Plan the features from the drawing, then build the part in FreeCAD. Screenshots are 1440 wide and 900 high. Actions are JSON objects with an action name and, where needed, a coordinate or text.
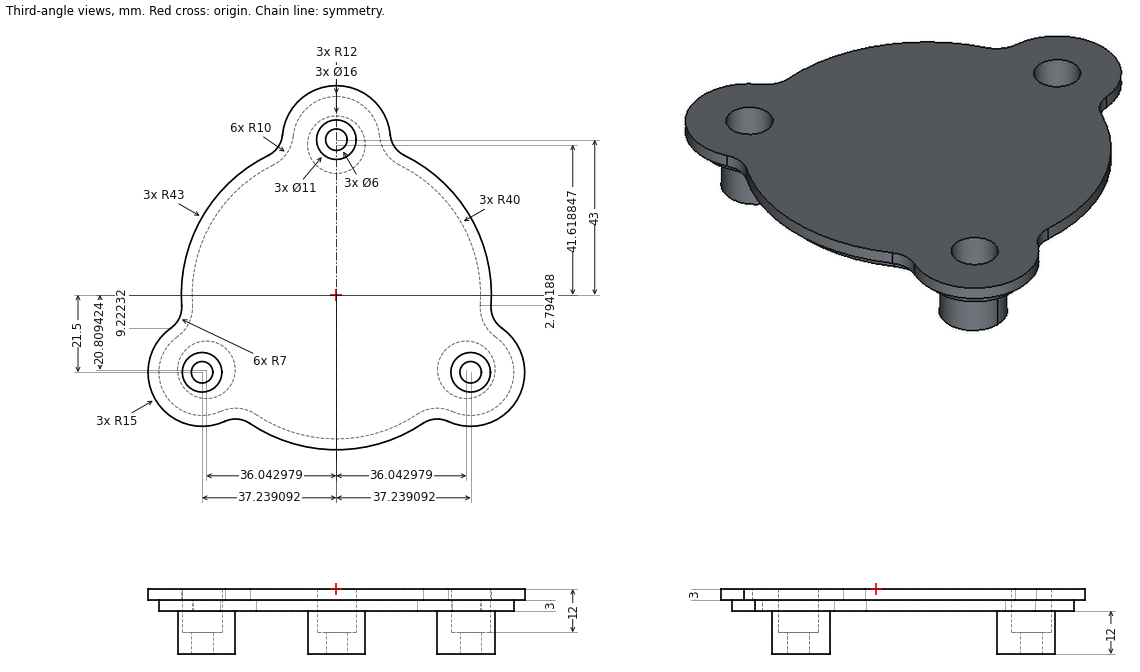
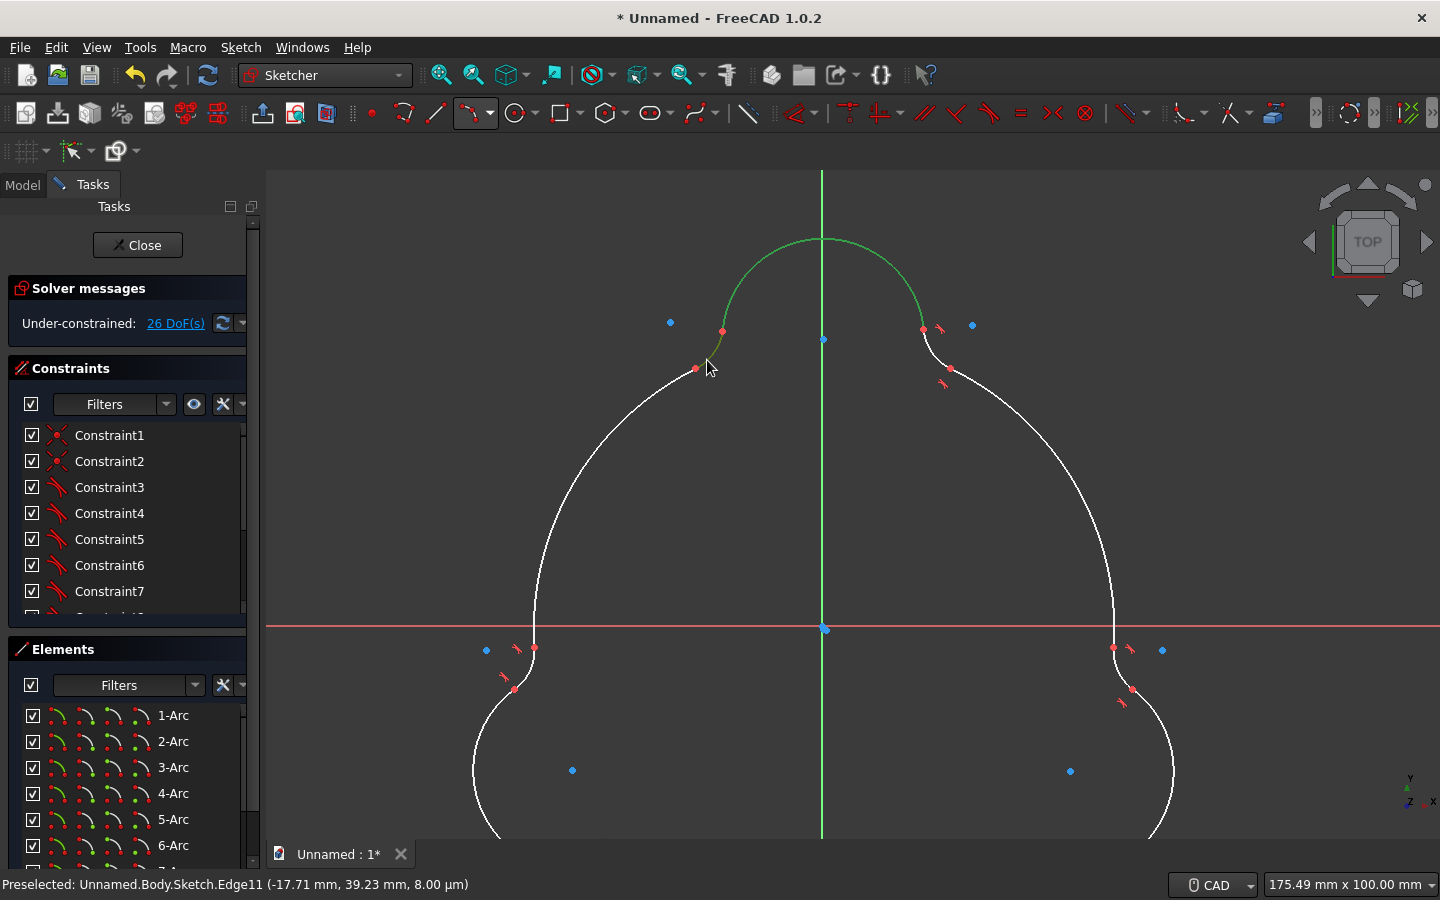
{"action": "left_click", "coordinate": [990, 114]}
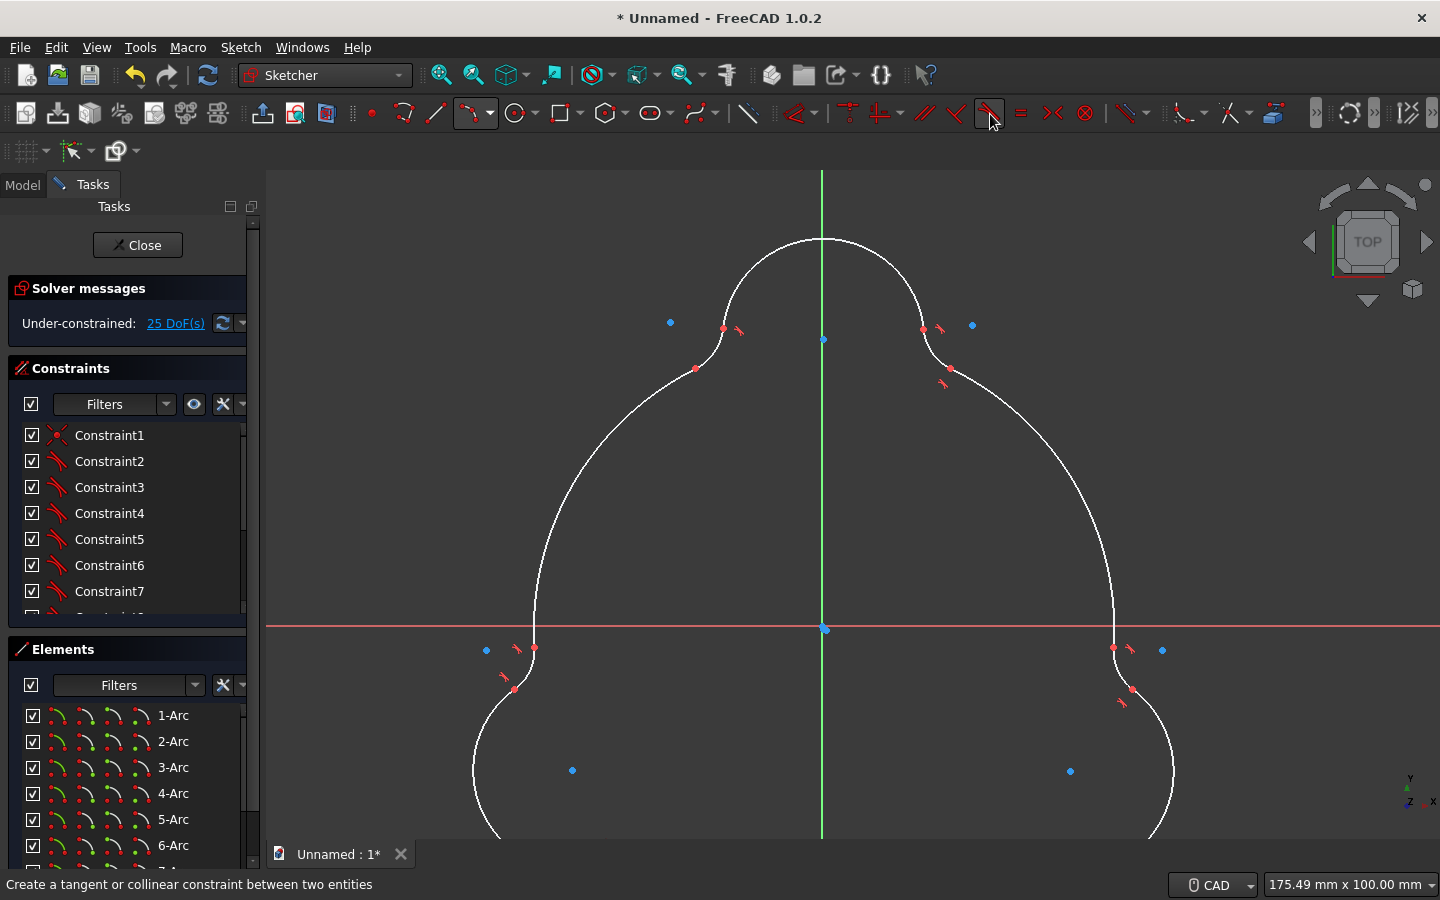
{"action": "left_click", "coordinate": [708, 360]}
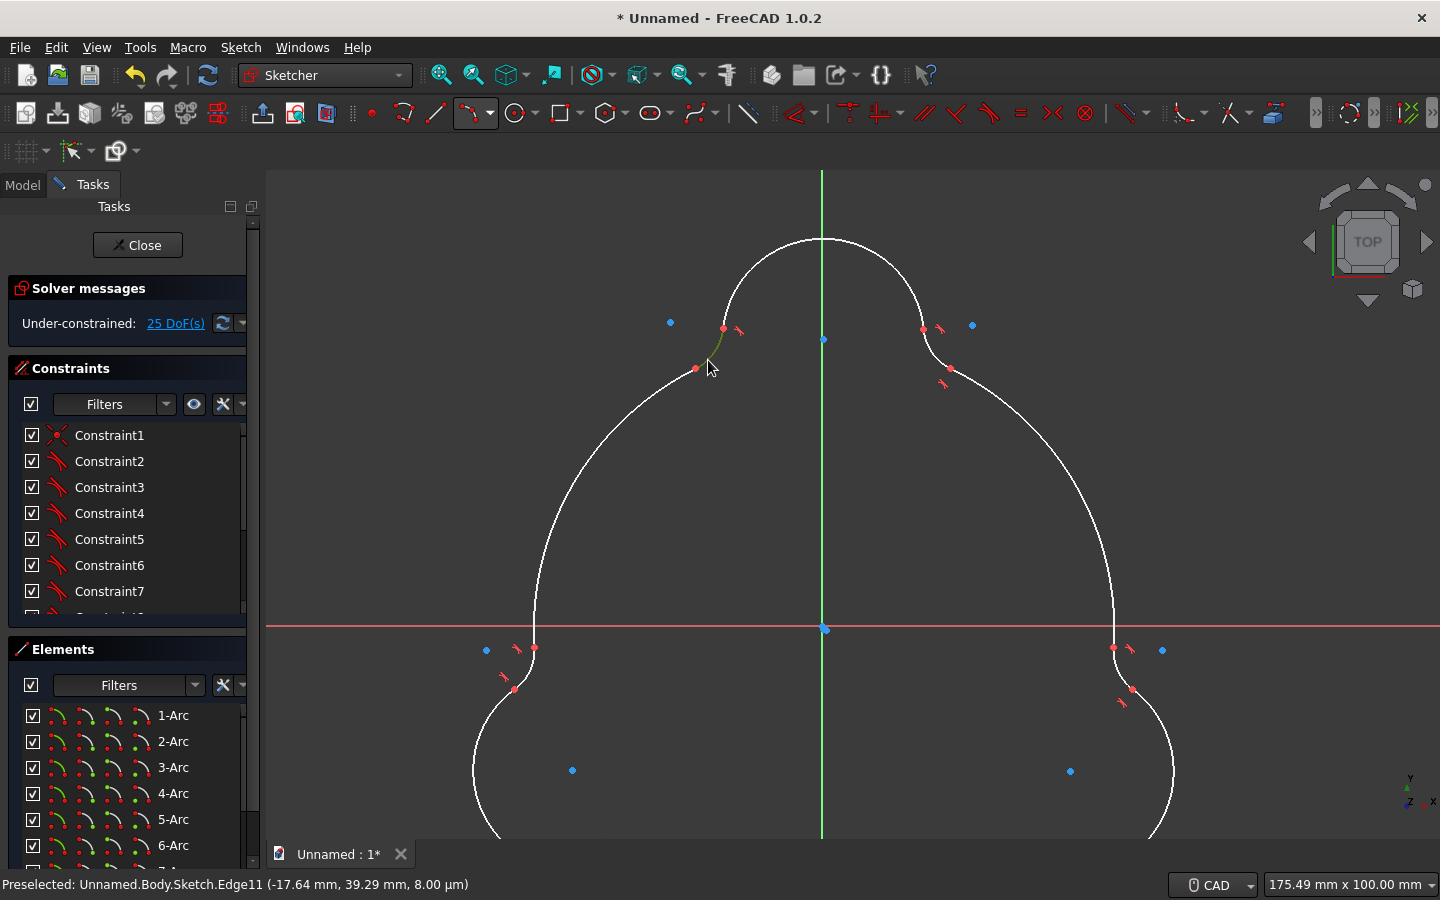
{"action": "left_click", "coordinate": [614, 429]}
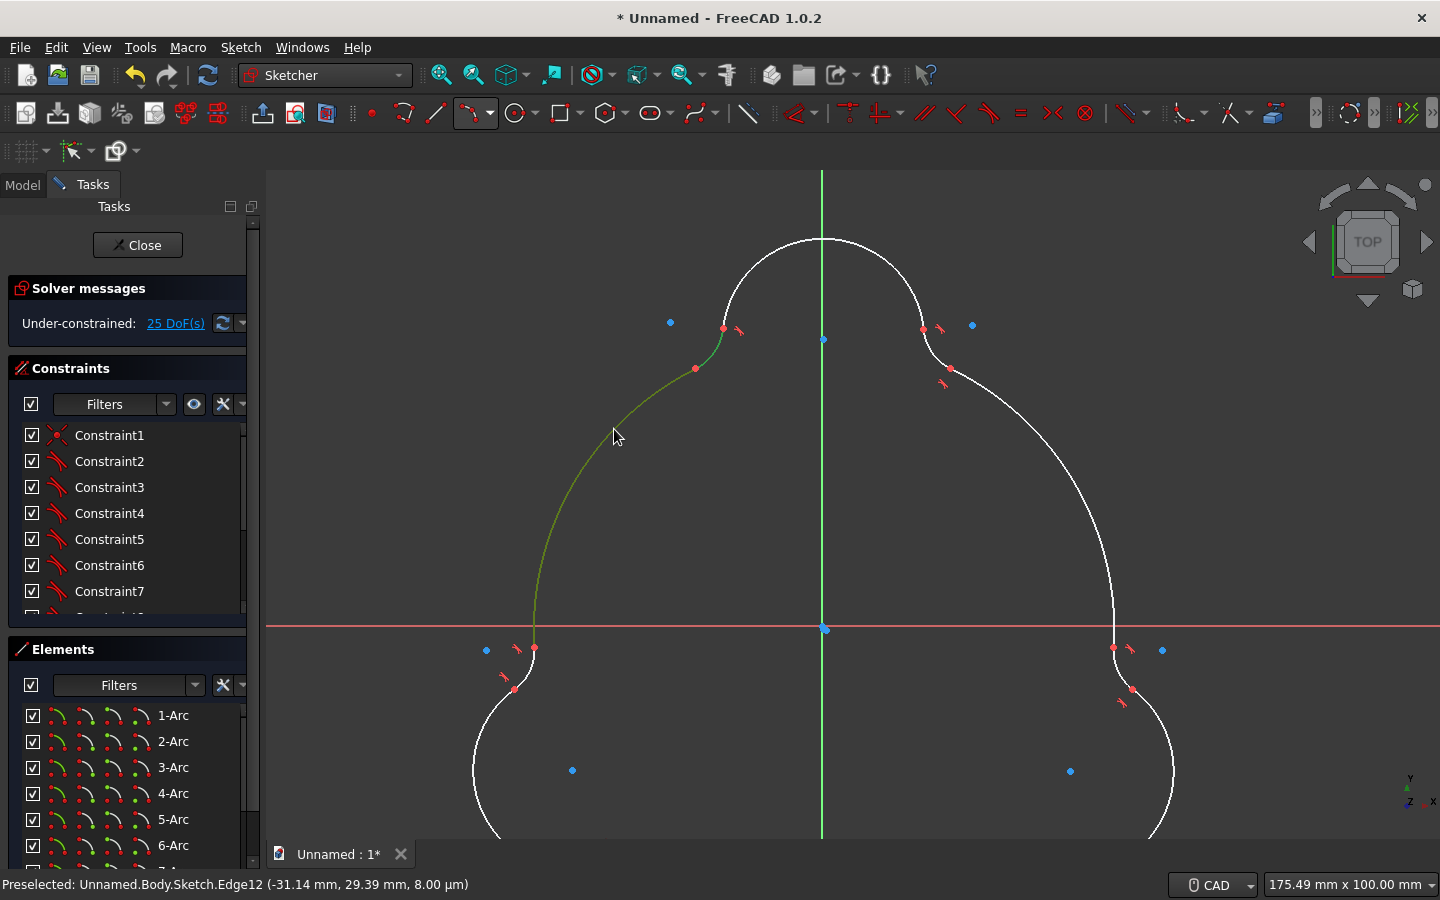
{"action": "left_click", "coordinate": [990, 114]}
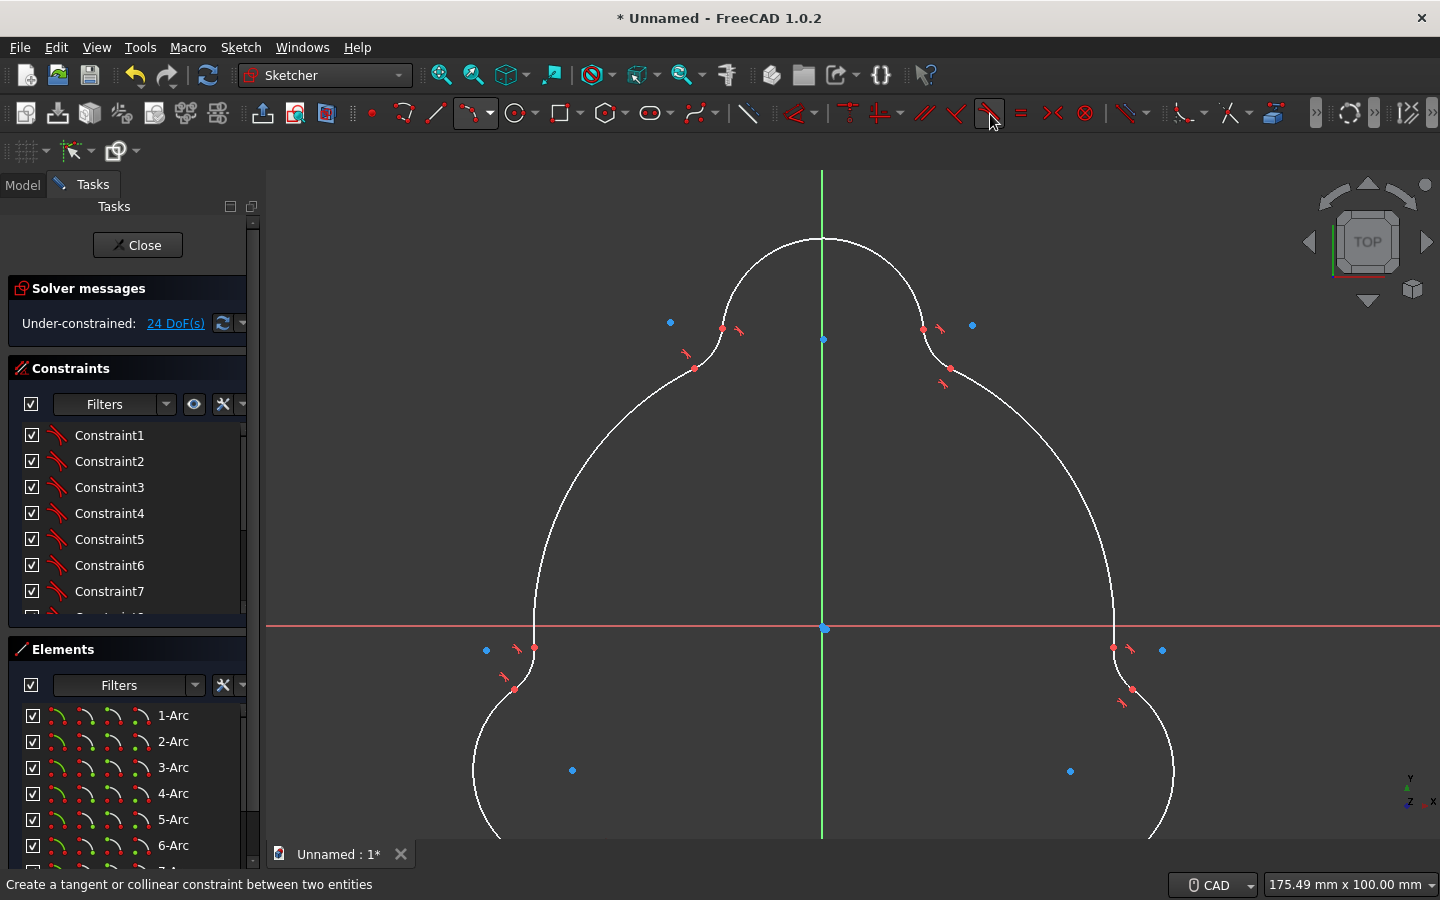
{"action": "scroll", "coordinate": [708, 359], "scroll_direction": "down", "scroll_amount": 2}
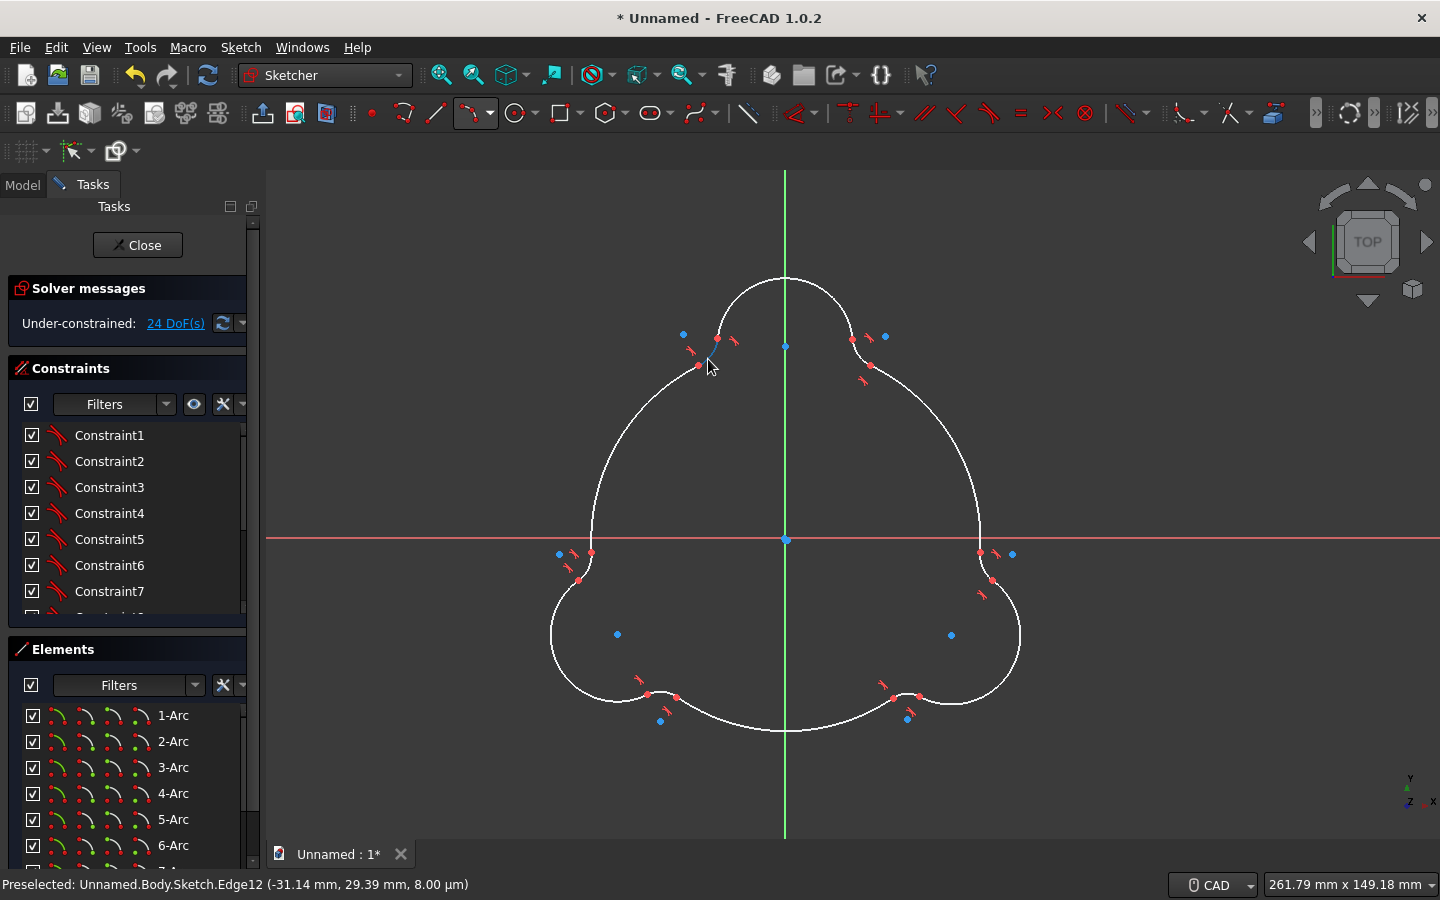
{"action": "left_click", "coordinate": [739, 725]}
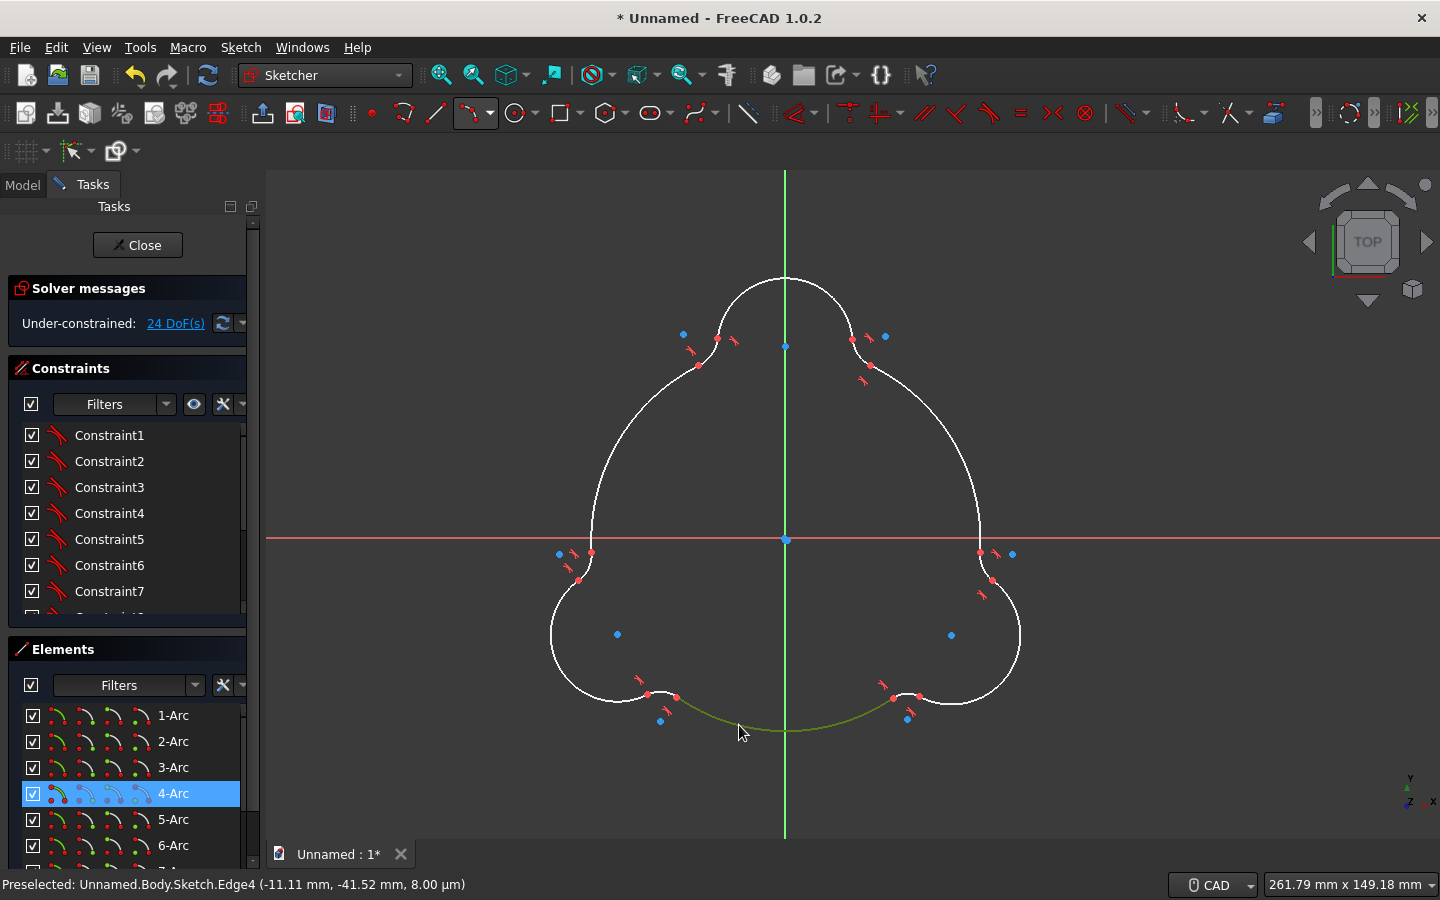
{"action": "left_click", "coordinate": [972, 485]}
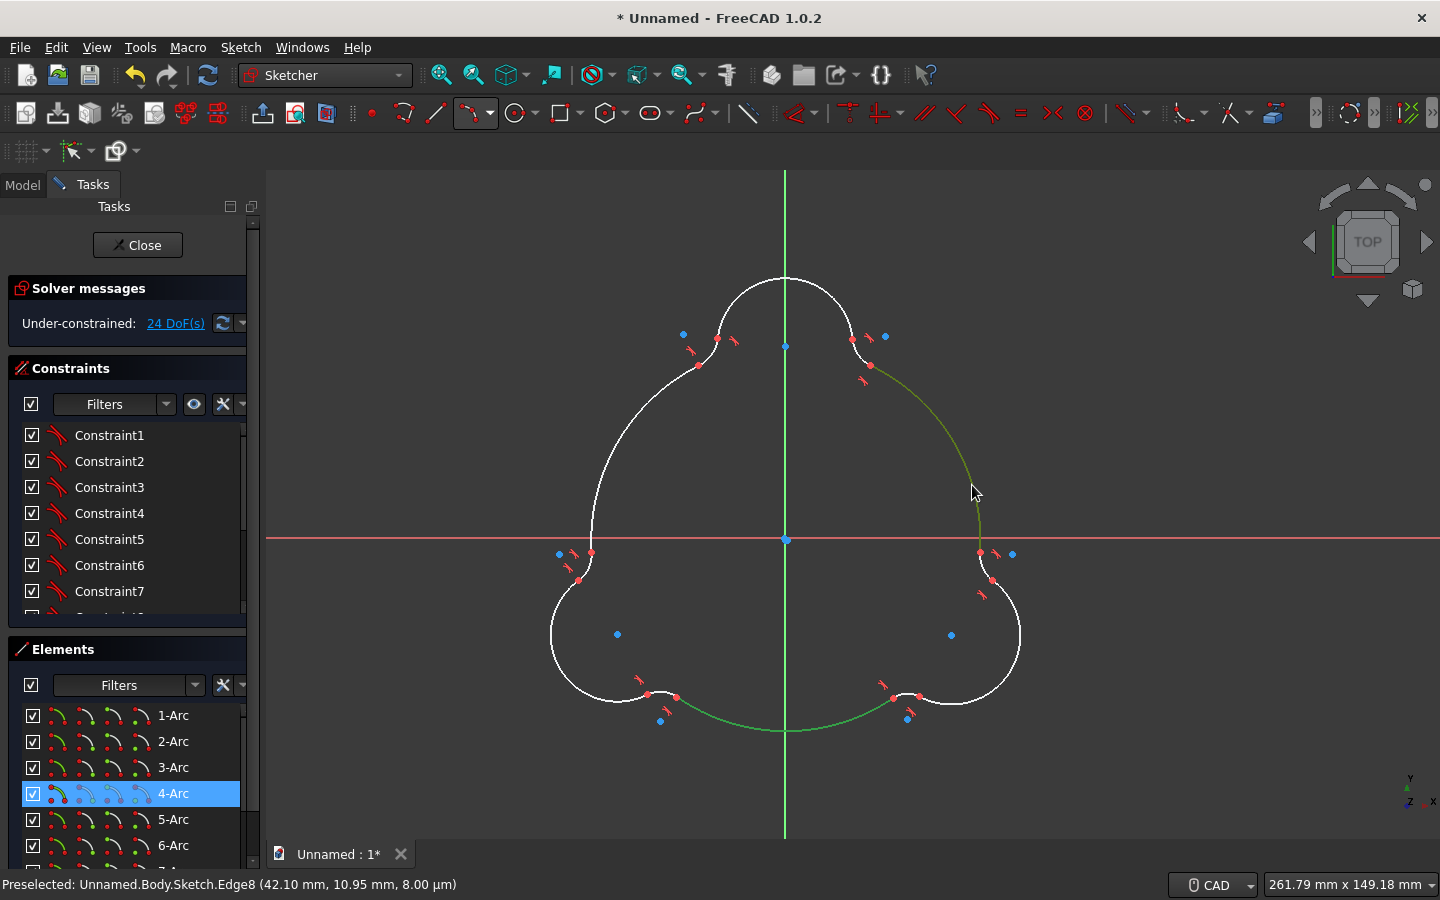
{"action": "left_click", "coordinate": [848, 114]}